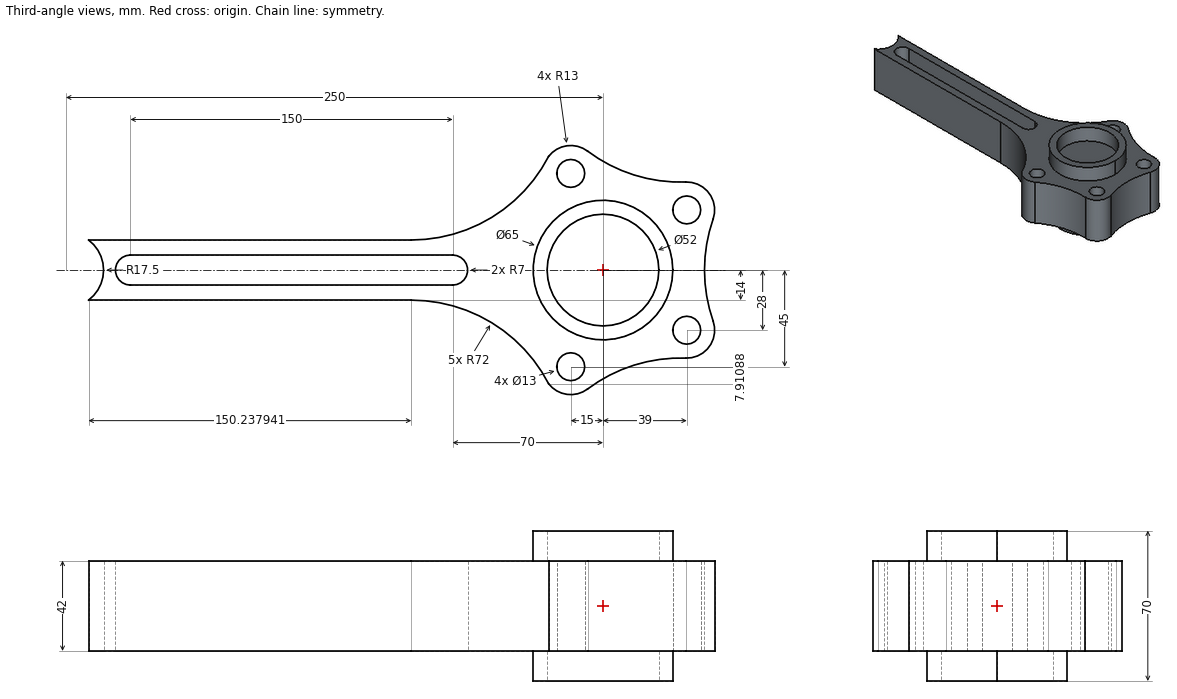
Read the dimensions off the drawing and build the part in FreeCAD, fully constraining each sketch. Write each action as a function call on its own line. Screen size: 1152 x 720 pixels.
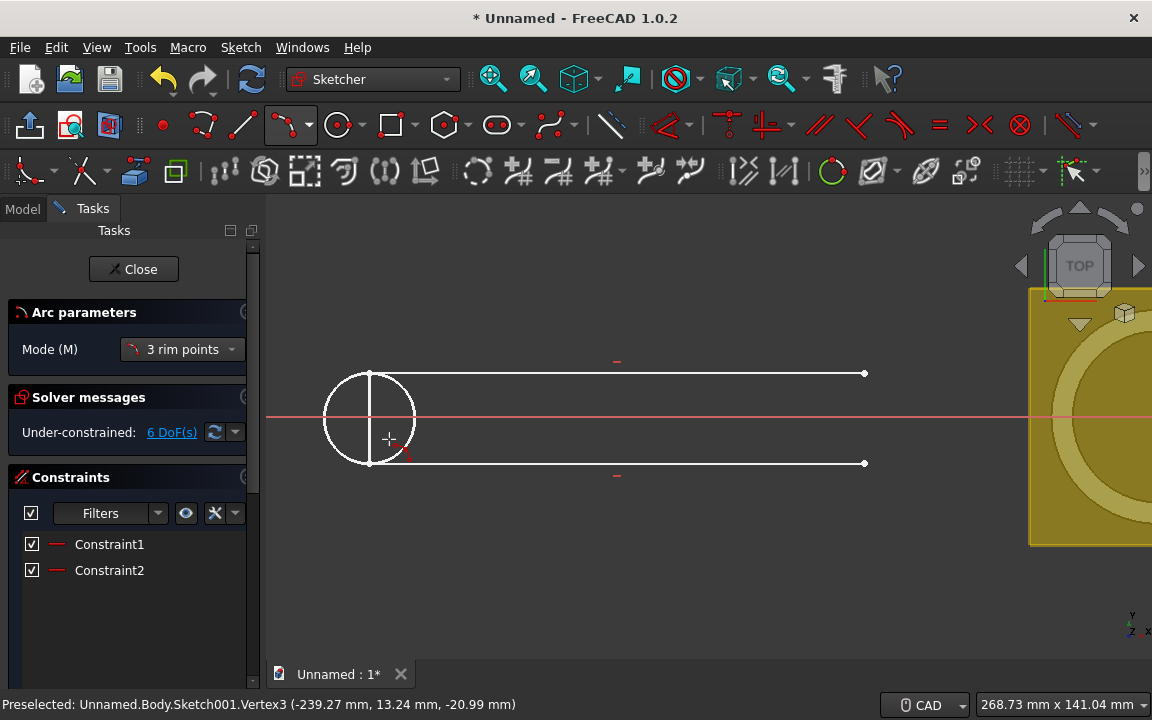
click(388, 438)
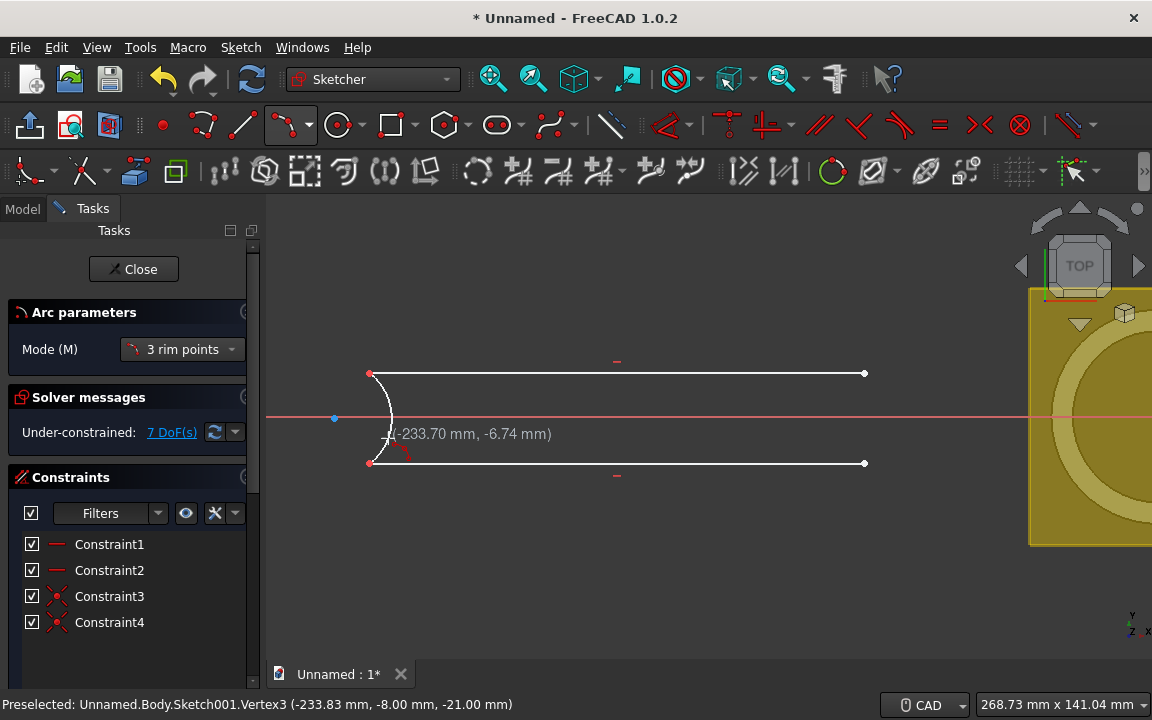
click(865, 373)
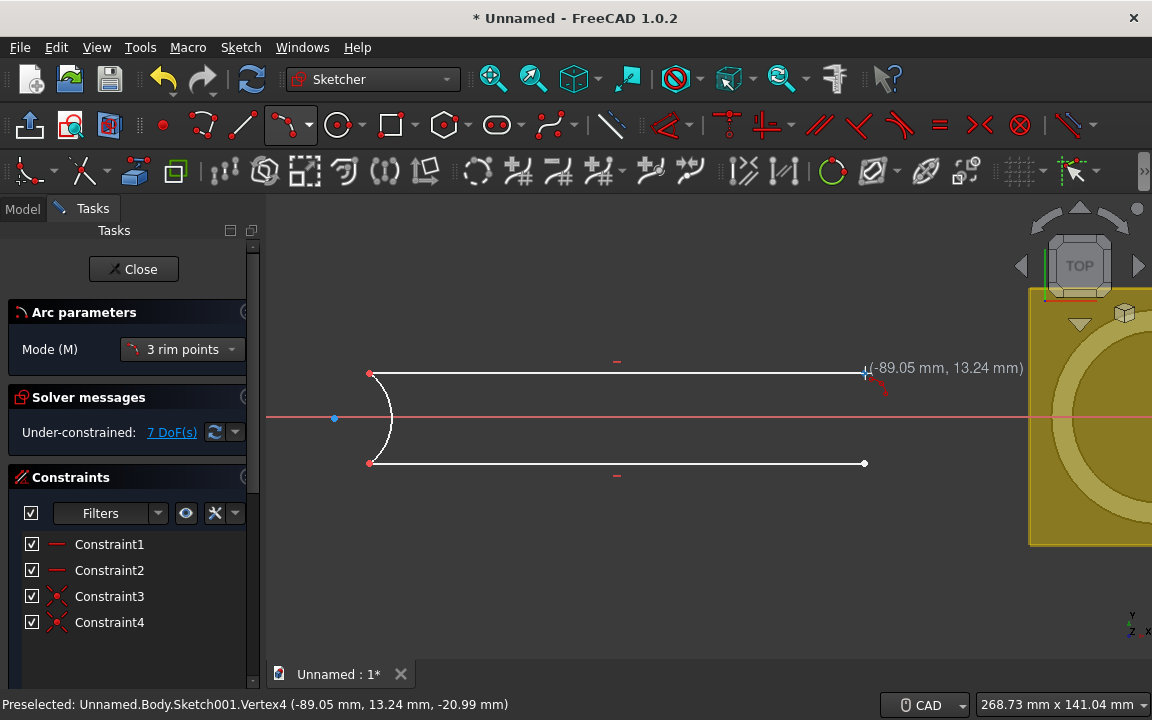
scroll(388, 438, down, 3)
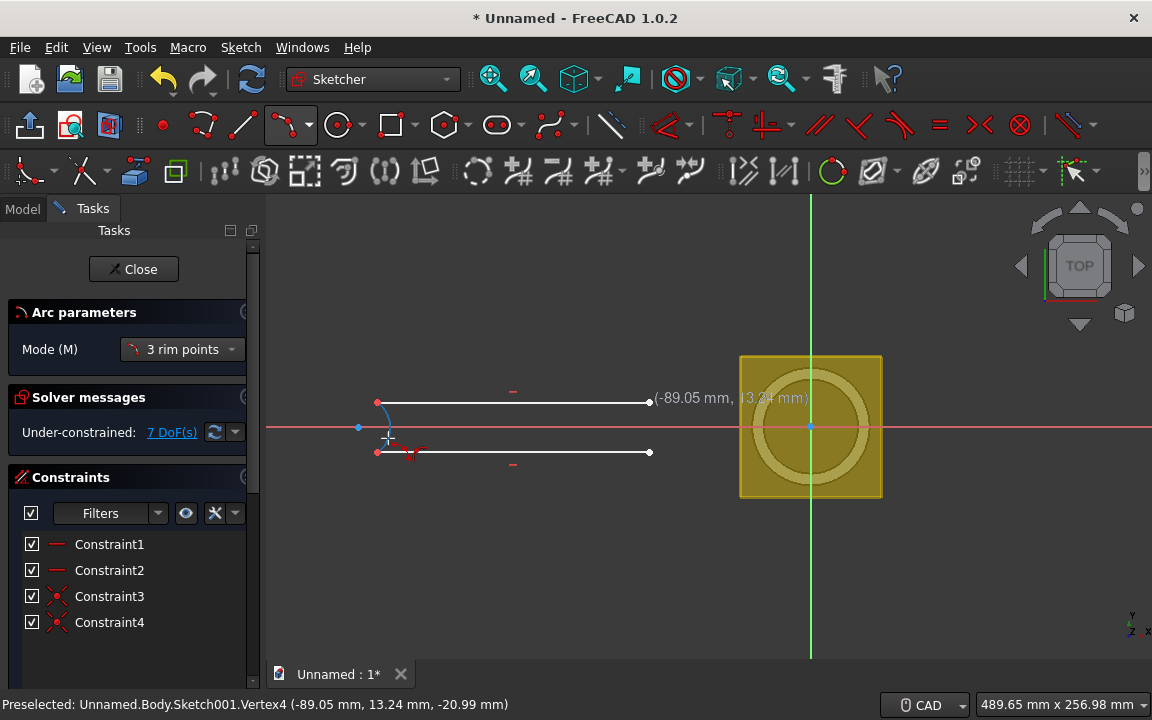
click(765, 331)
click(717, 382)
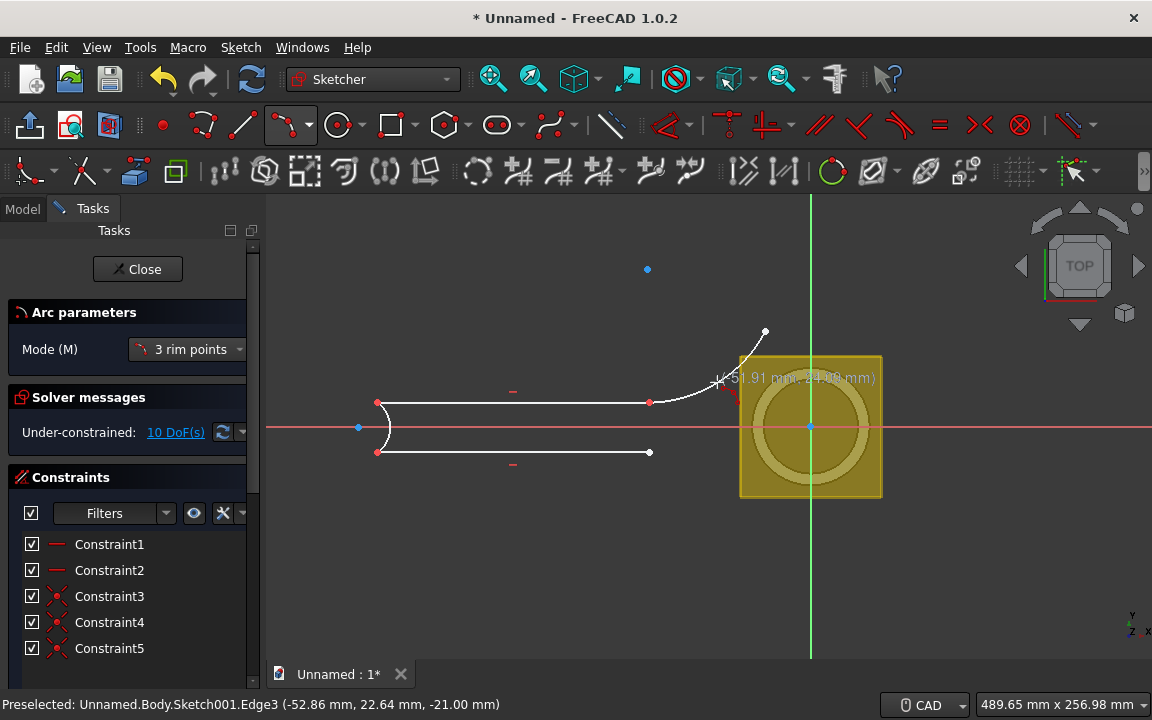
click(765, 332)
click(798, 326)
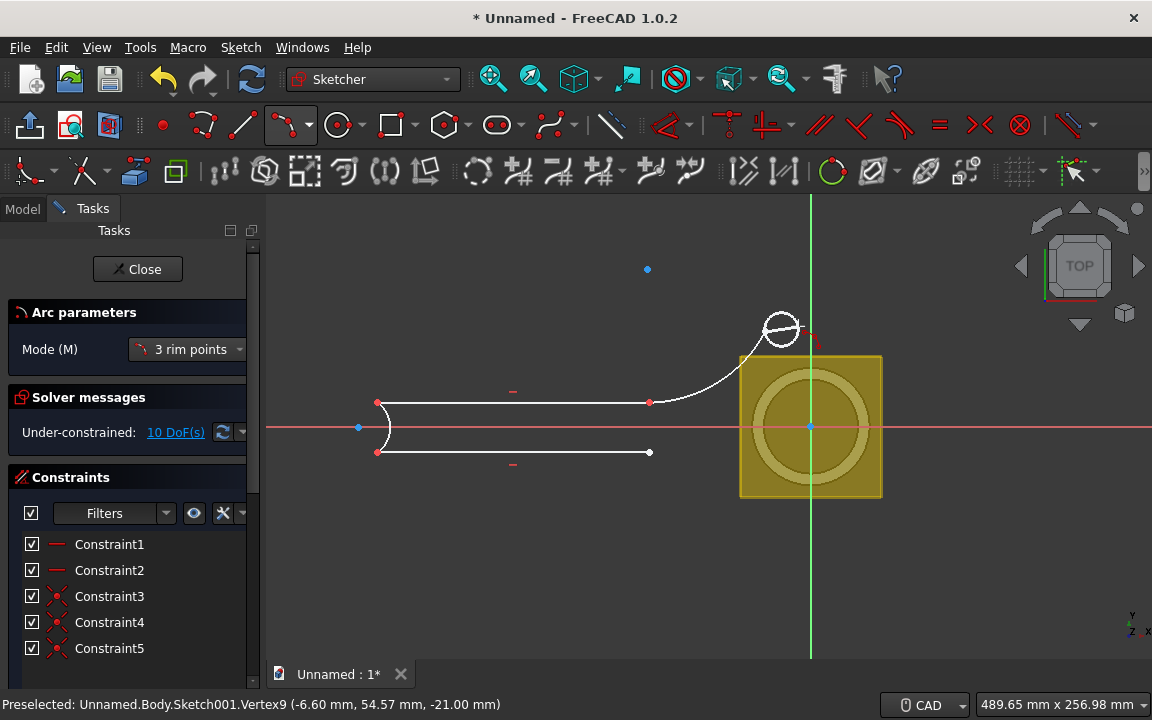
scroll(781, 322, up, 5)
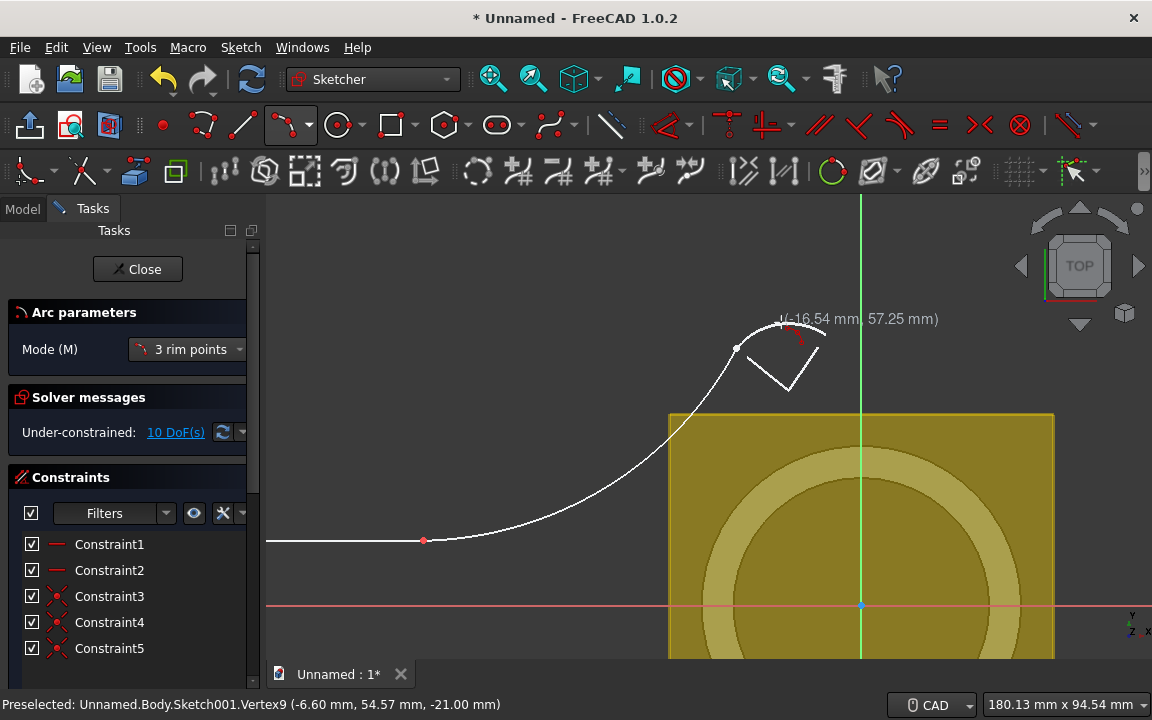
click(779, 321)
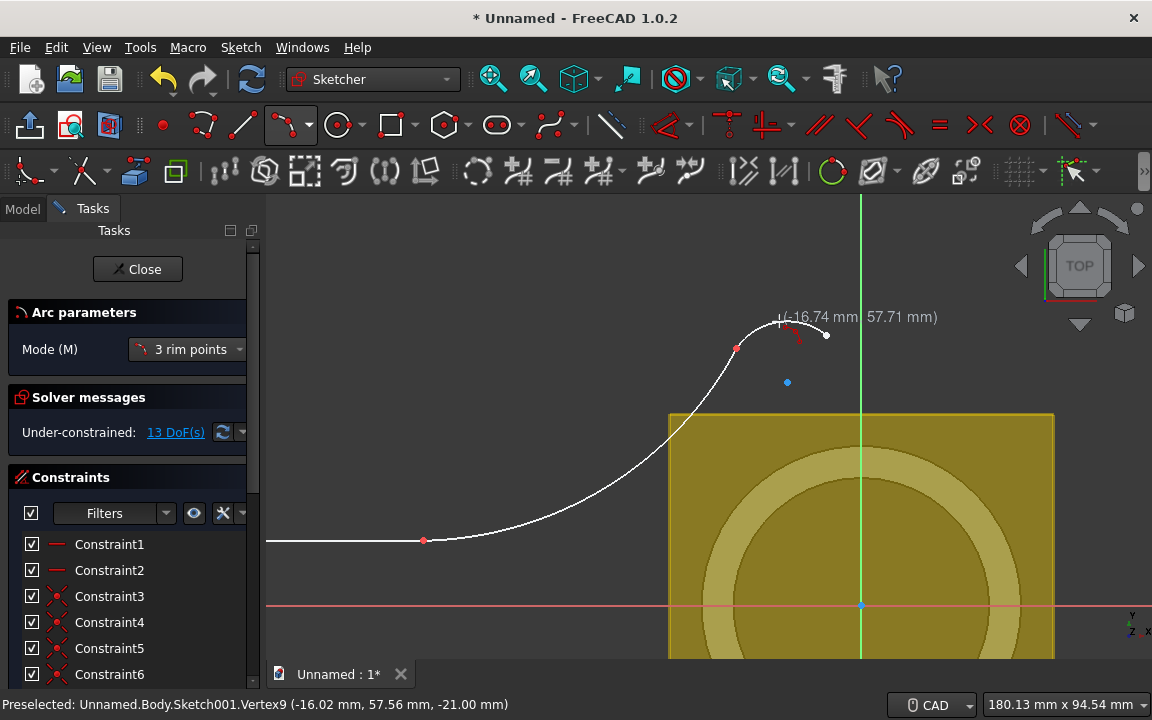
click(826, 335)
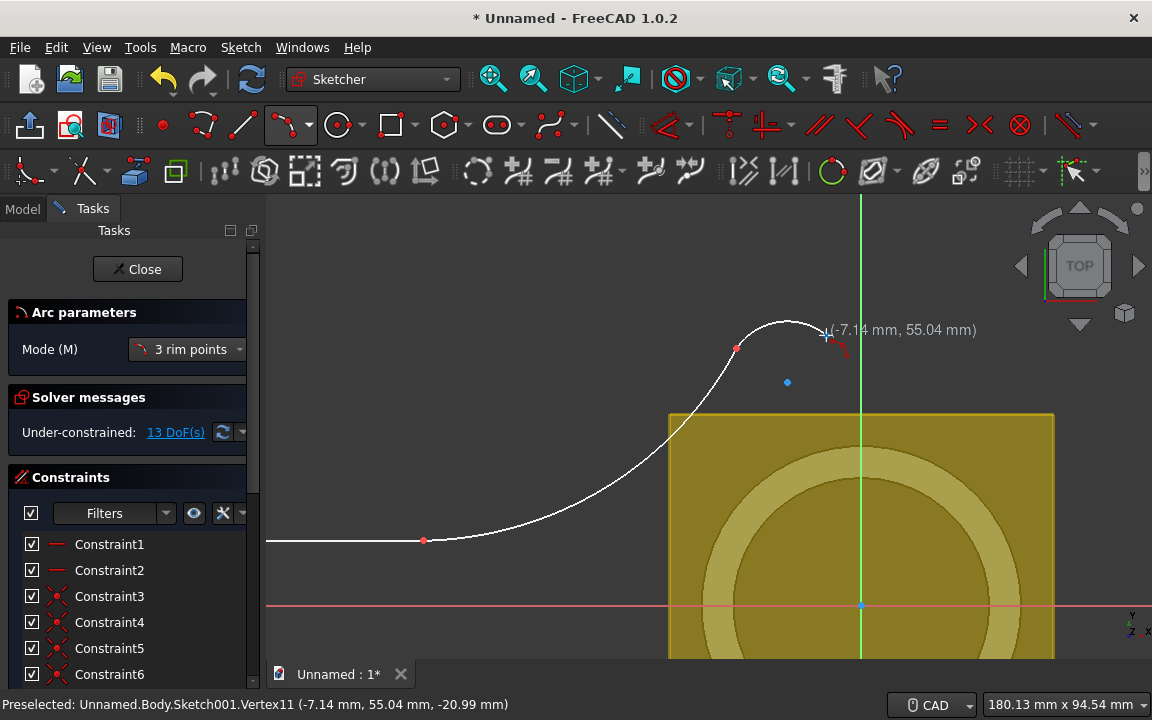
scroll(781, 322, down, 5)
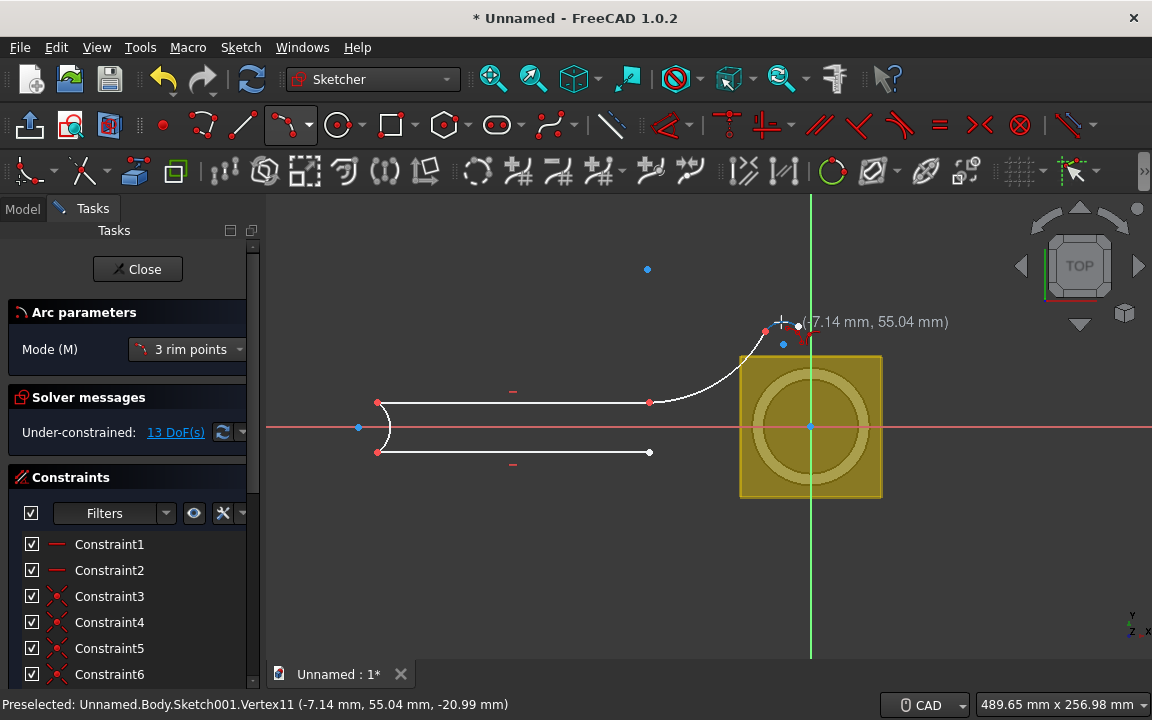
click(881, 352)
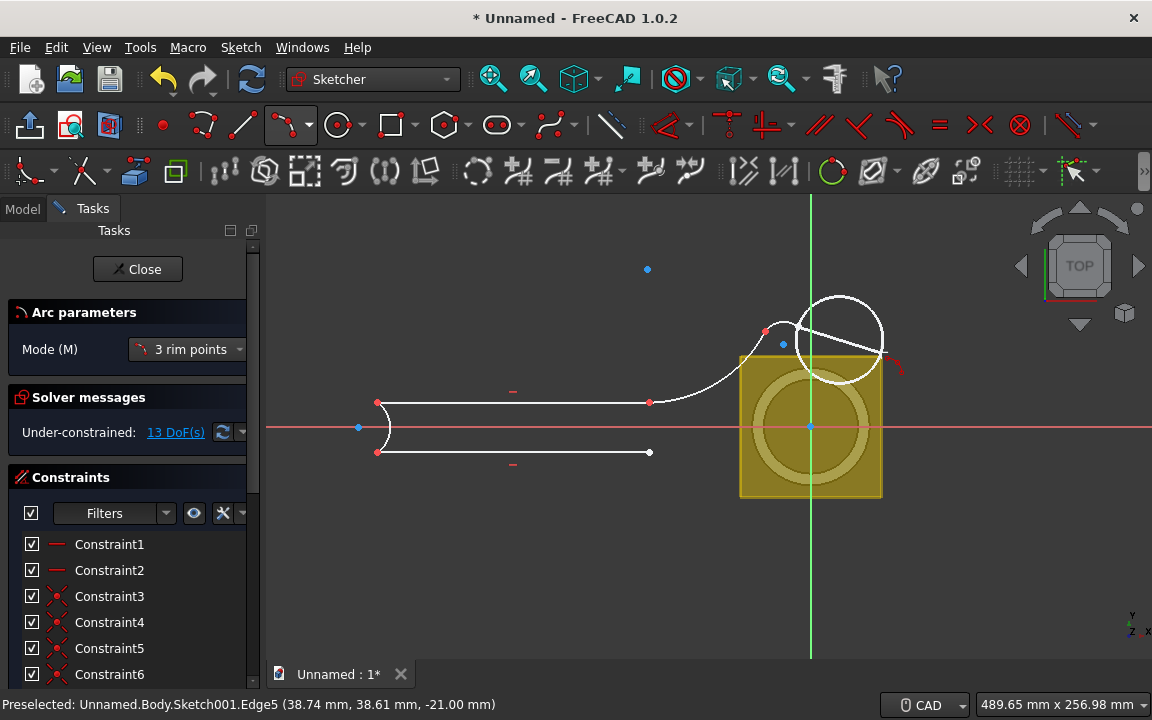
scroll(837, 346, up, 4)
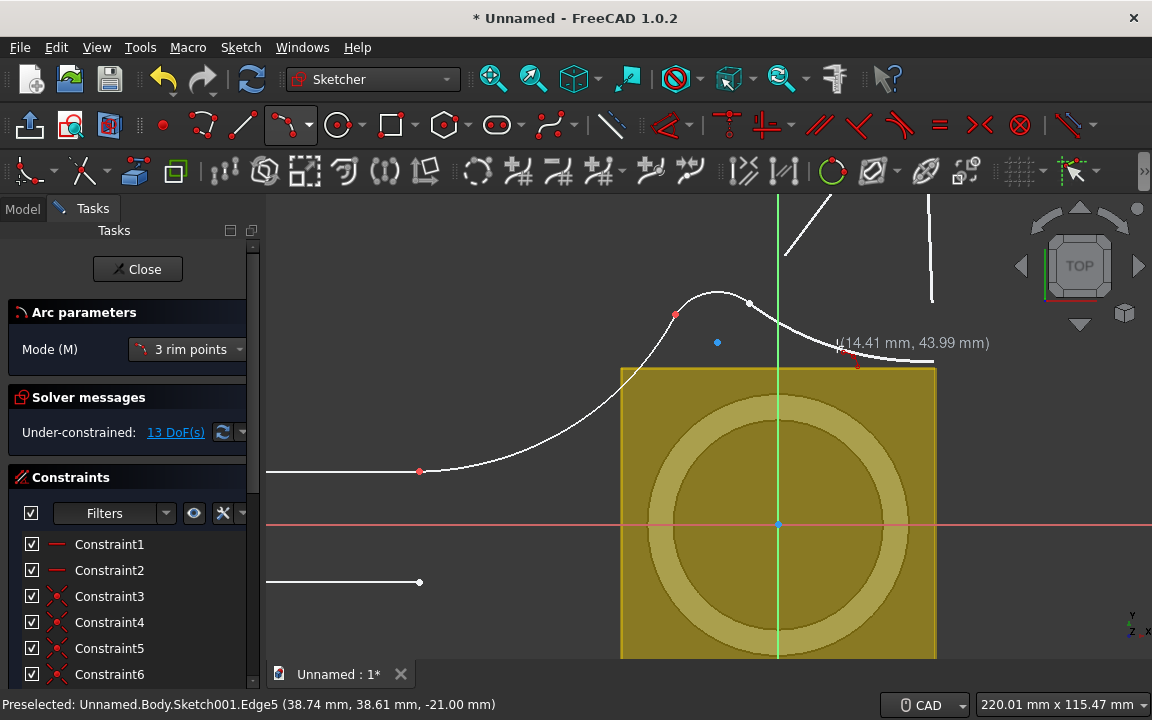
click(836, 347)